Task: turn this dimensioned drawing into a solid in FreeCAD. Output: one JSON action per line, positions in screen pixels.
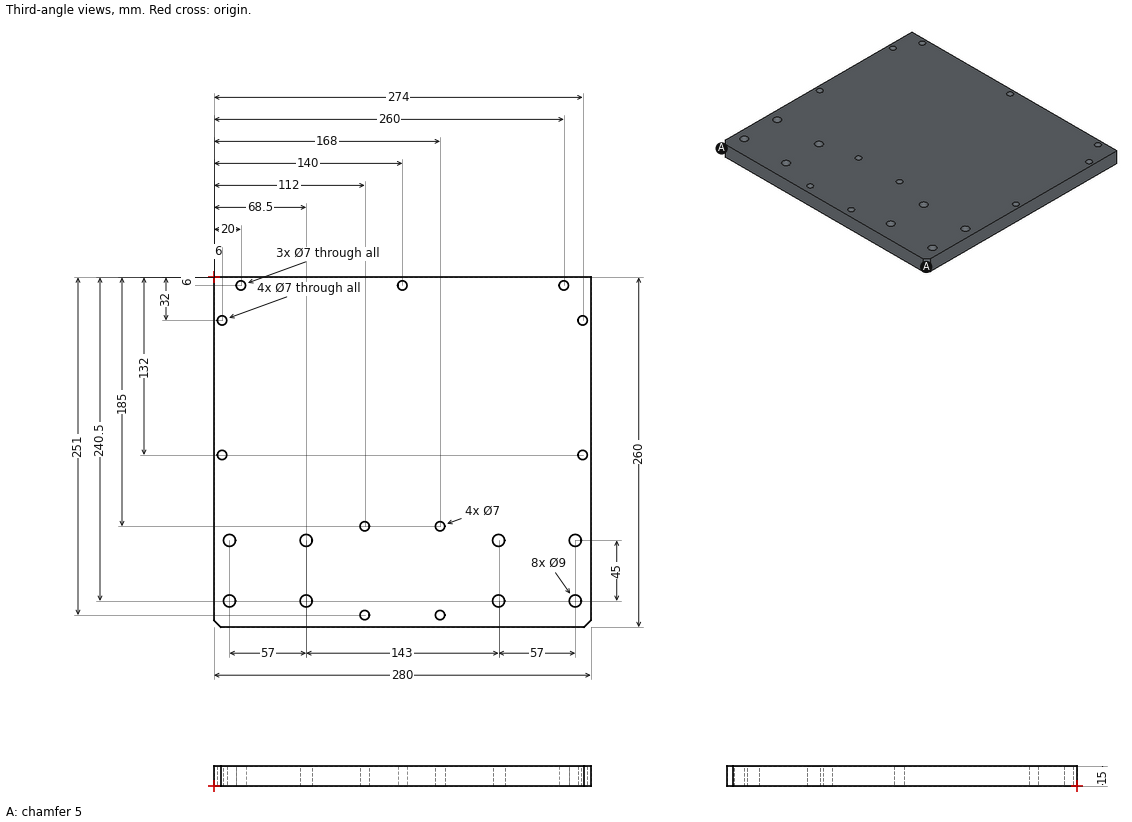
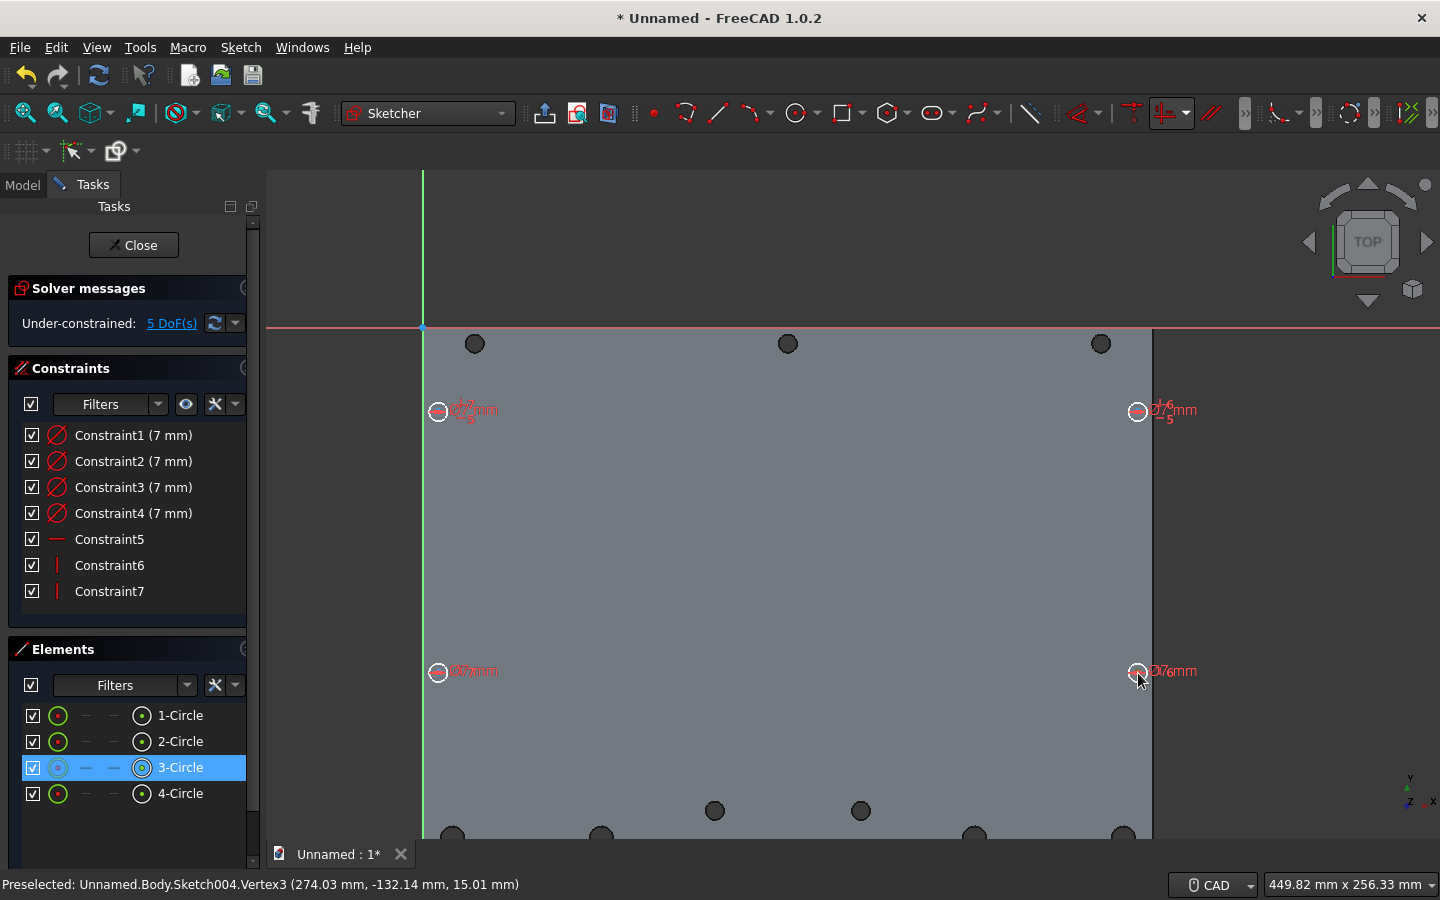
{"action": "left_click", "coordinate": [438, 673]}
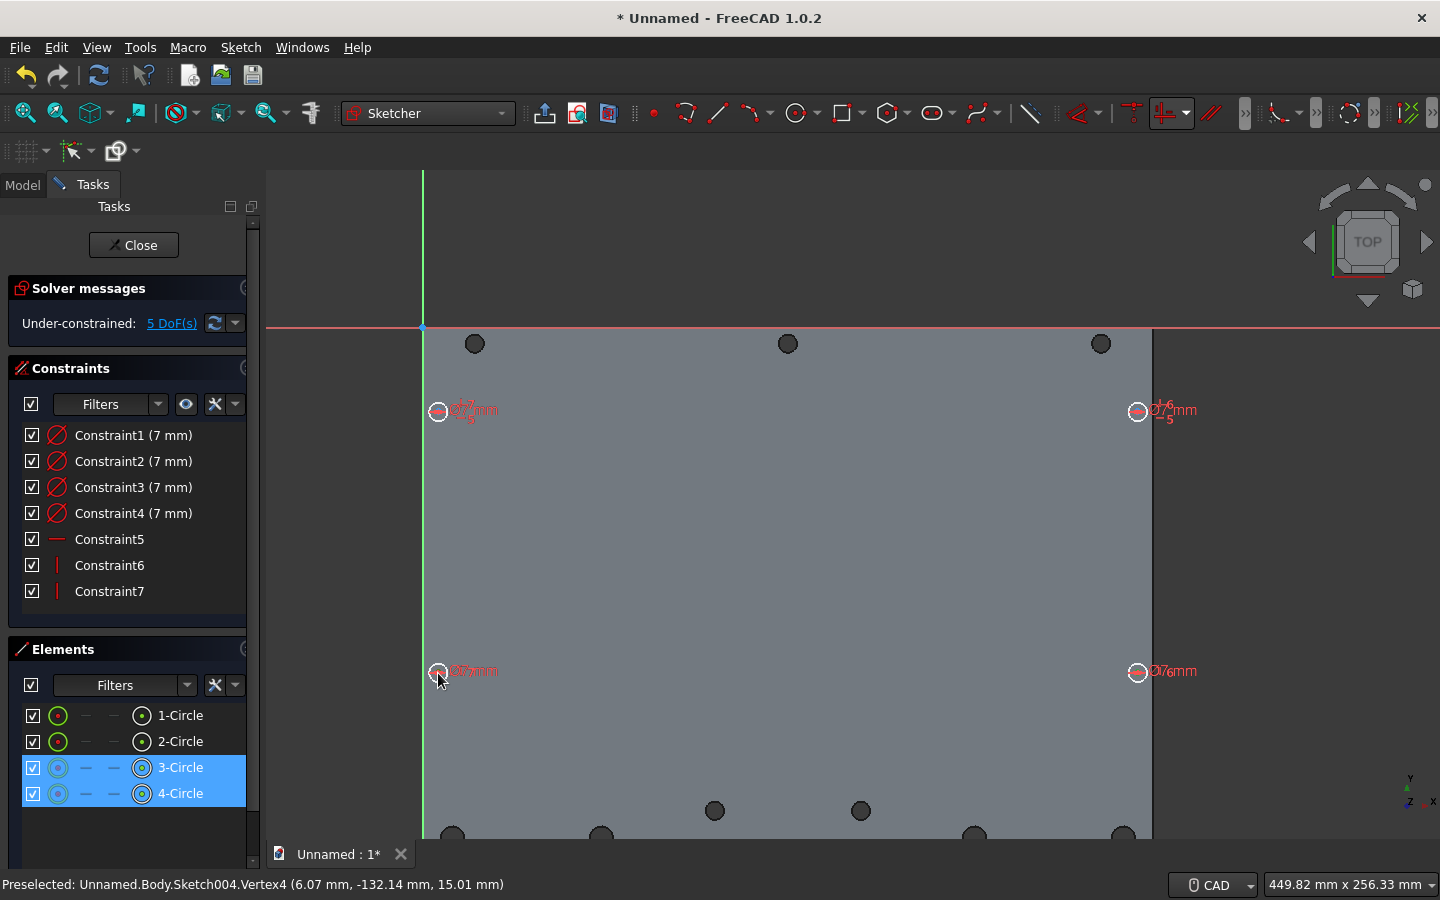
{"action": "key", "text": "h"}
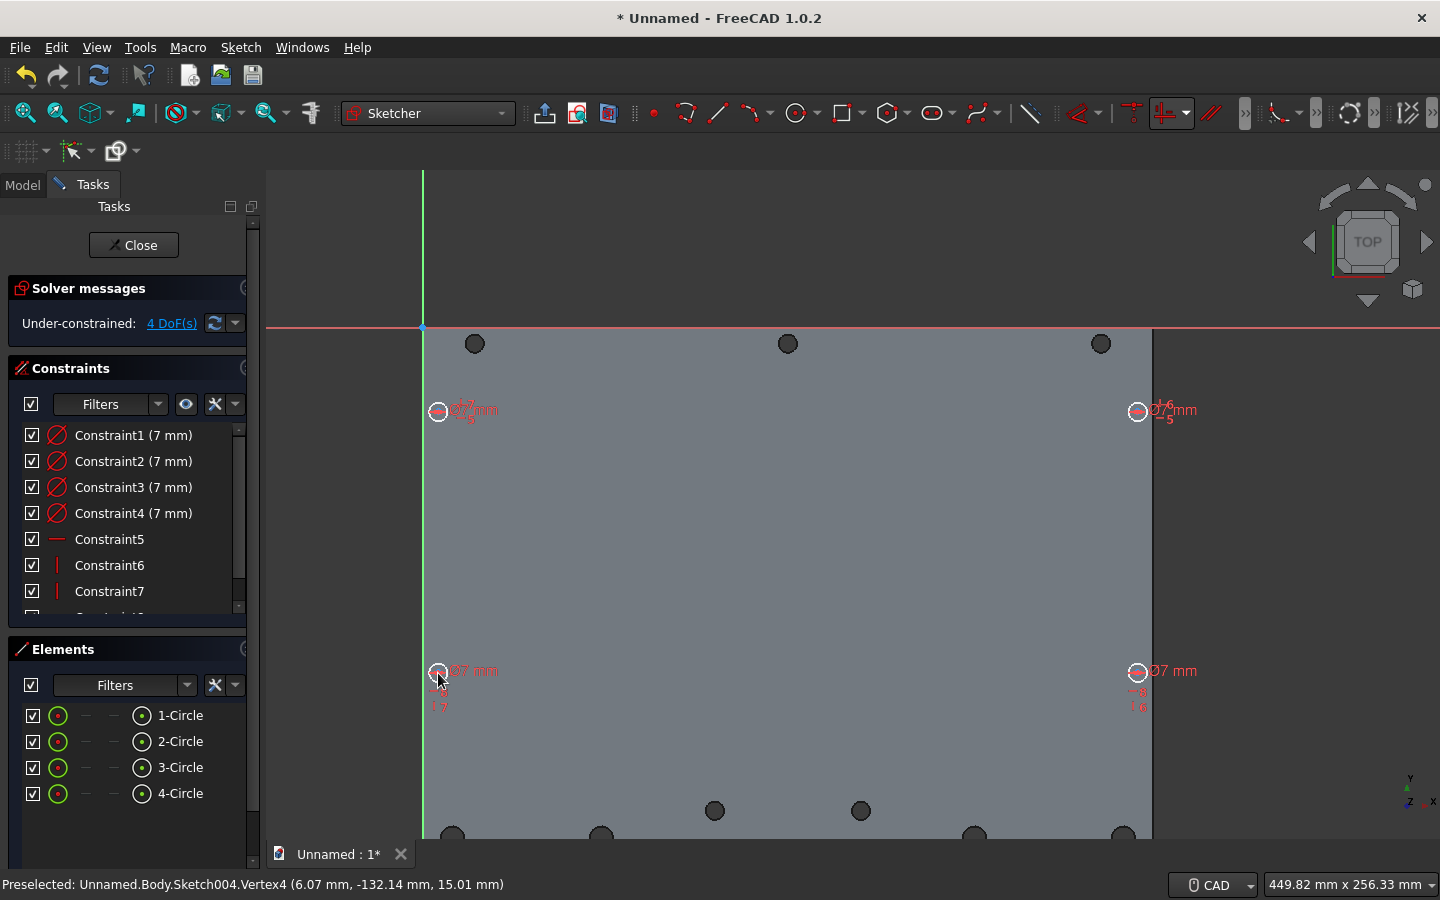
{"action": "left_click", "coordinate": [1078, 114]}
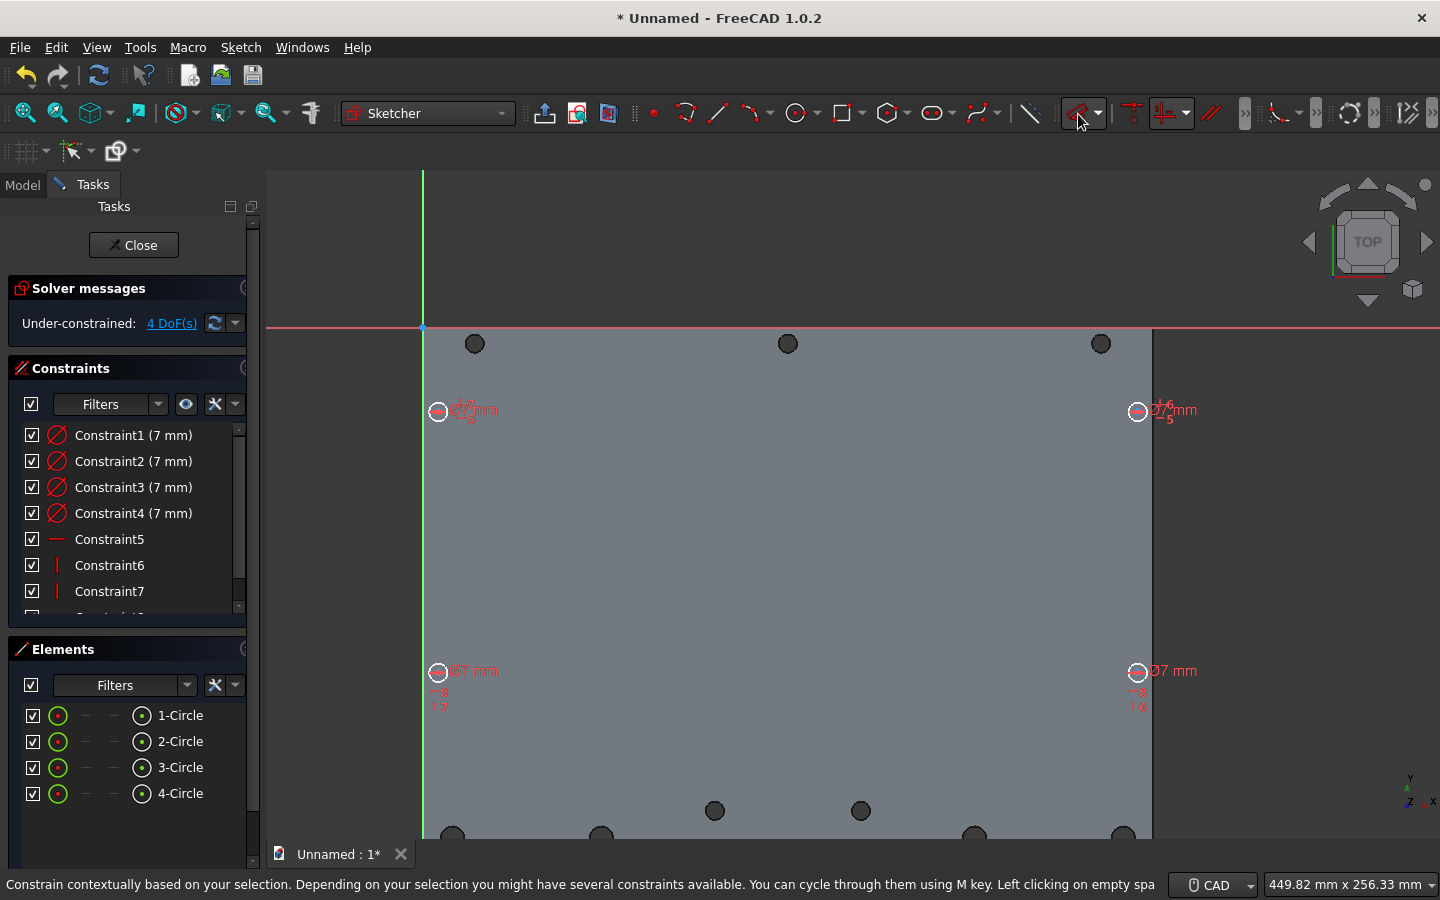
{"action": "scroll", "coordinate": [438, 412], "scroll_direction": "up", "scroll_amount": 5}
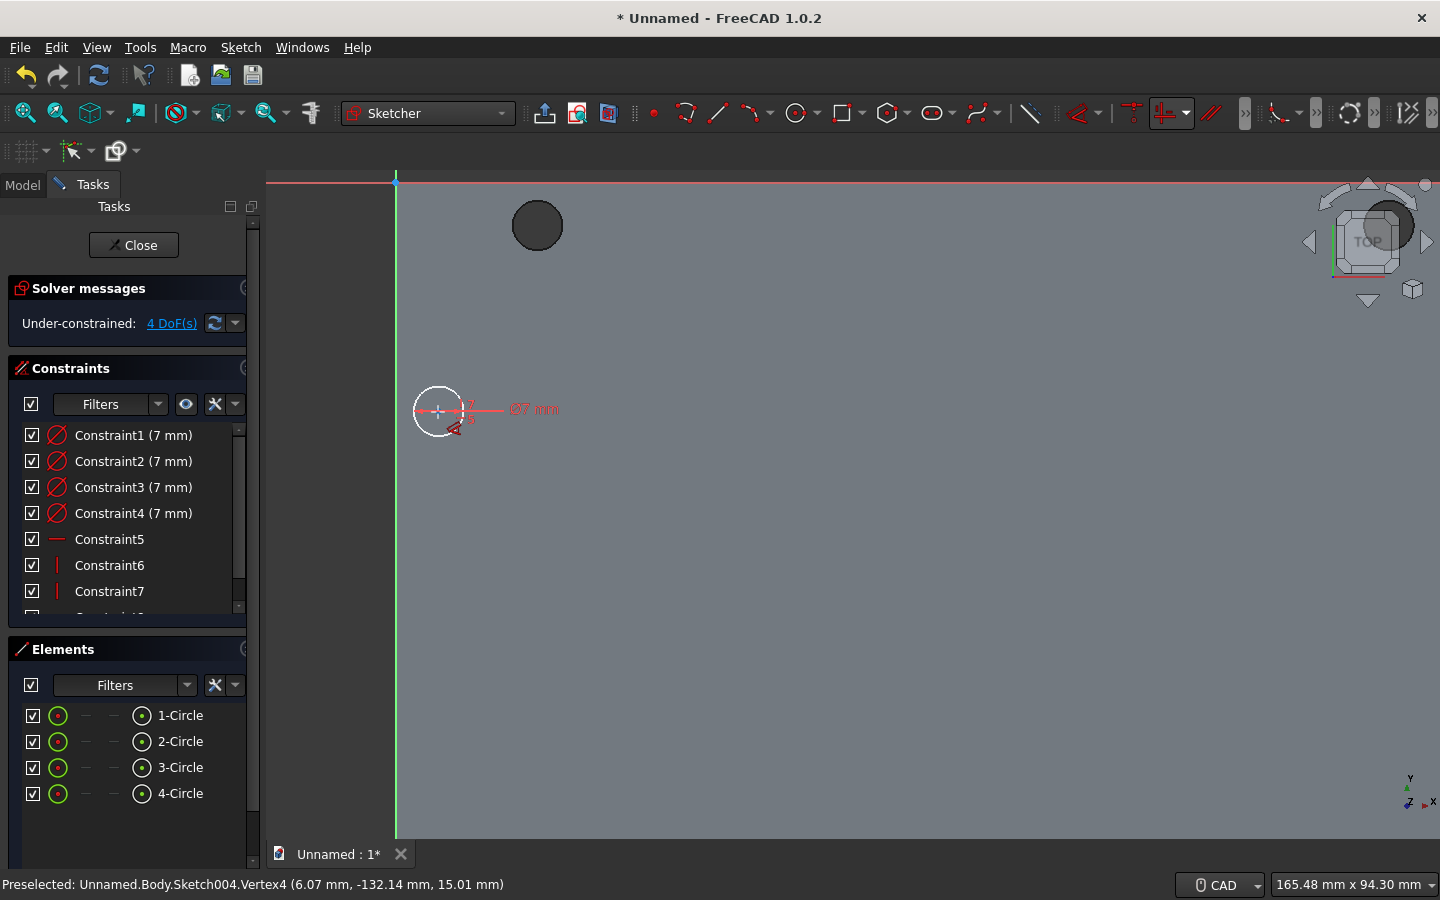
{"action": "left_click", "coordinate": [439, 411]}
{"action": "left_click", "coordinate": [417, 445]}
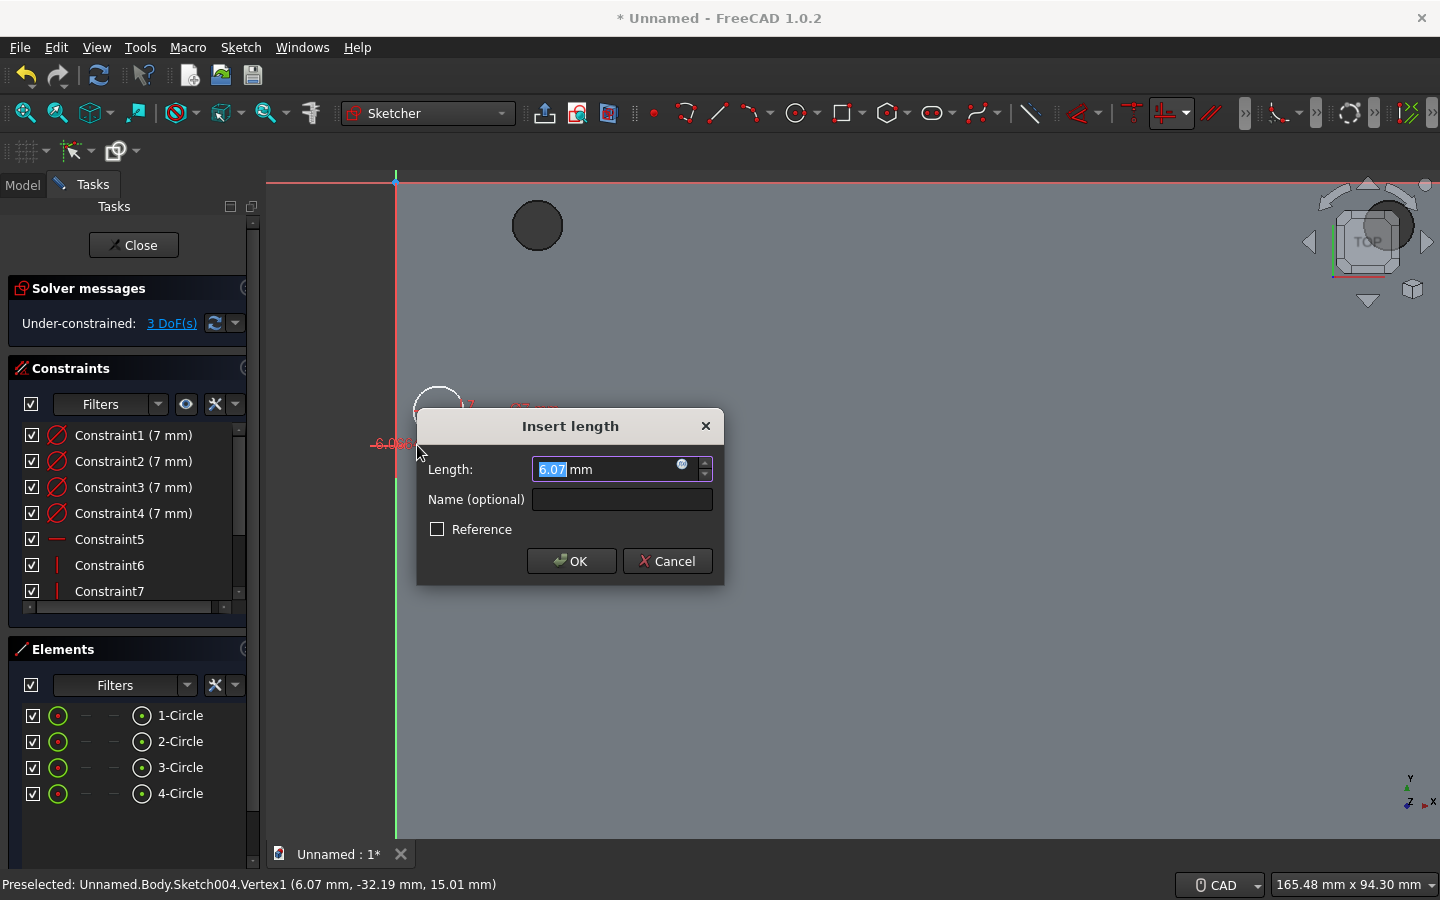
{"action": "type", "text": "6"}
{"action": "key", "text": "Return"}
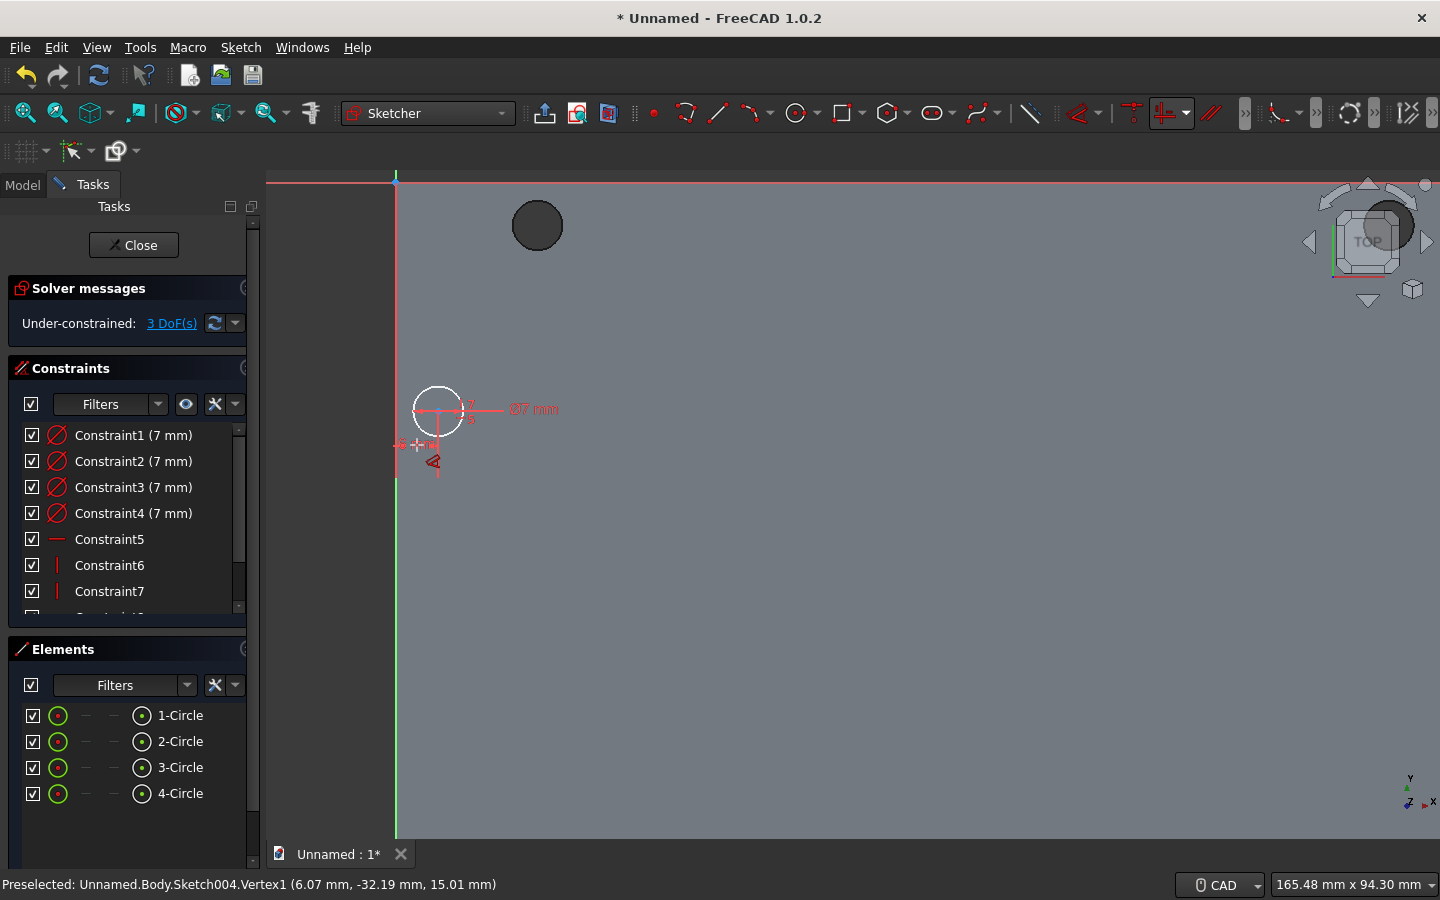
{"action": "left_click", "coordinate": [438, 411]}
{"action": "left_click", "coordinate": [362, 305]}